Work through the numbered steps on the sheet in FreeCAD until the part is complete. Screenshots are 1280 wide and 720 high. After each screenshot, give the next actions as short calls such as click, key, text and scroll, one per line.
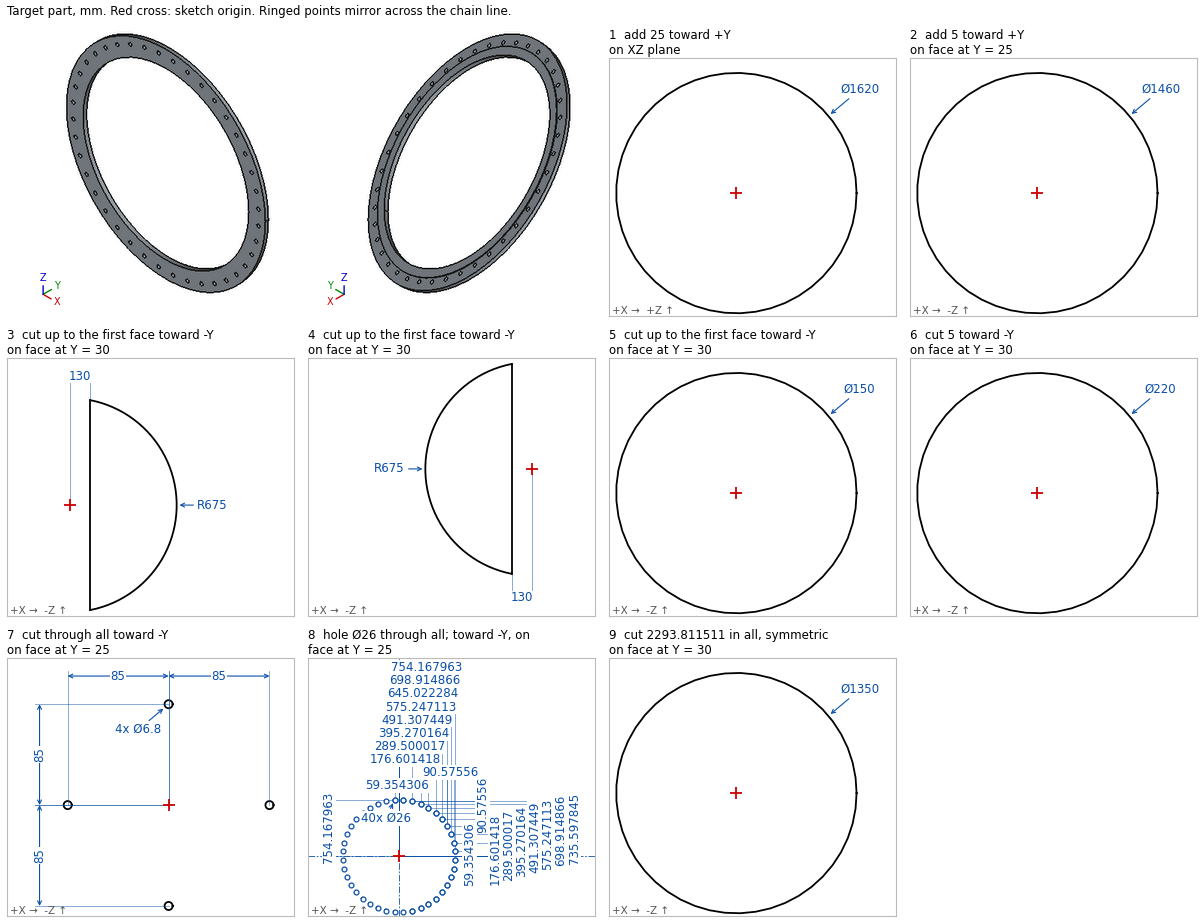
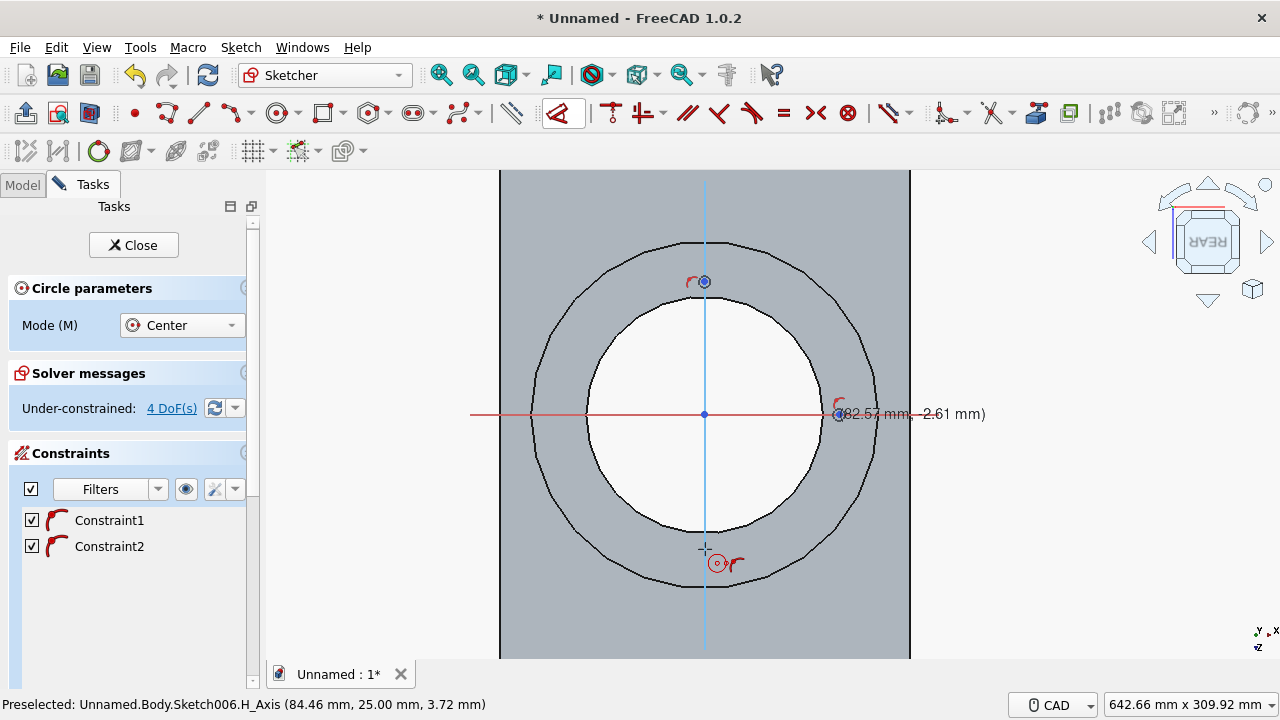
click(705, 549)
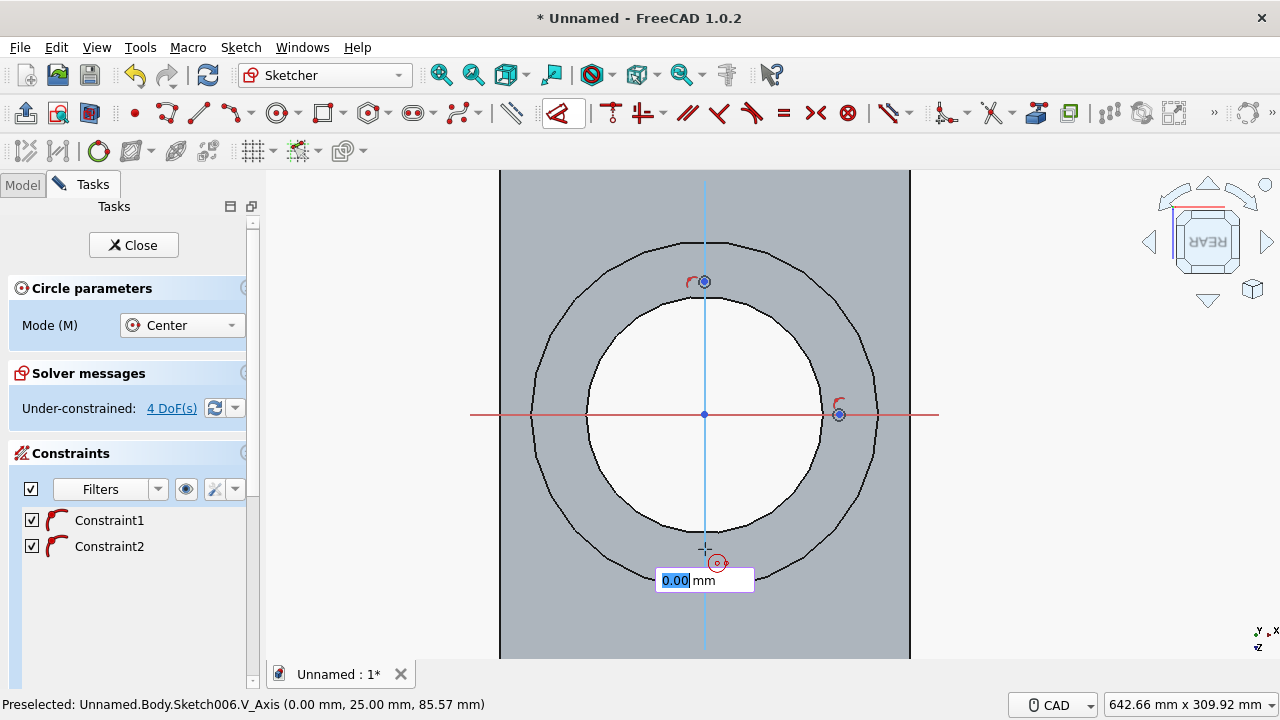
scroll(710, 547, up, 6)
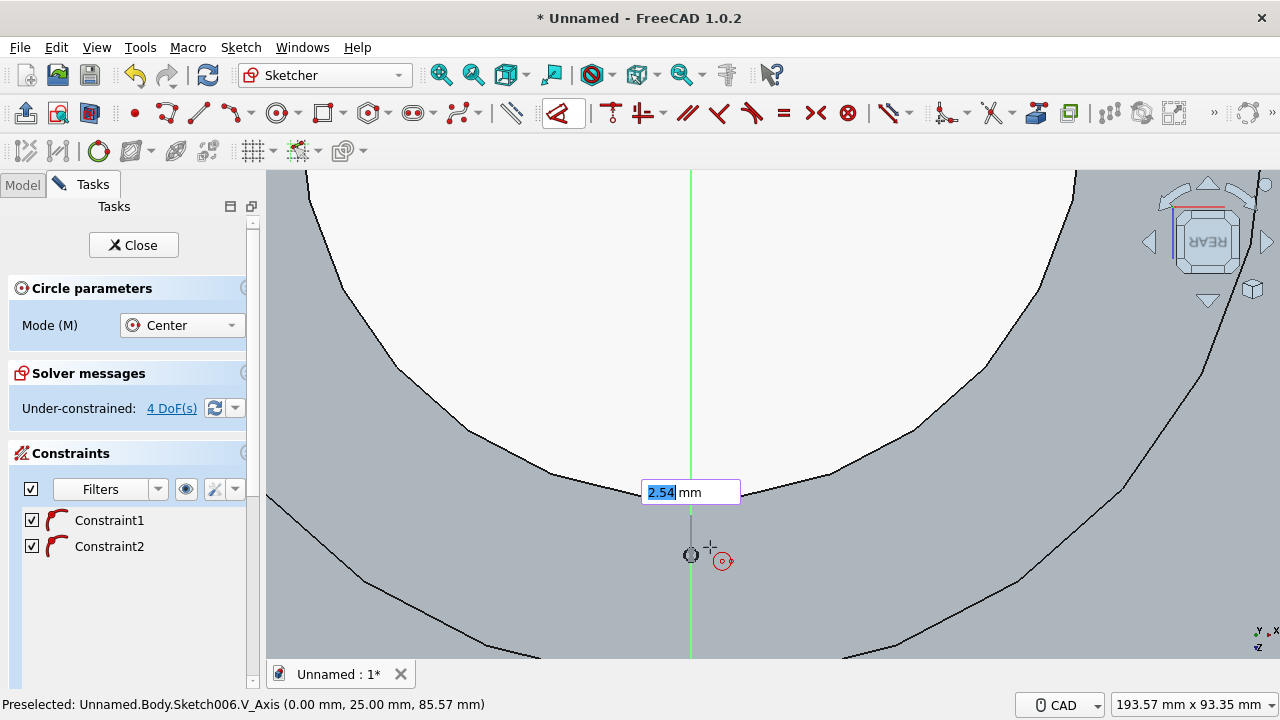
click(708, 546)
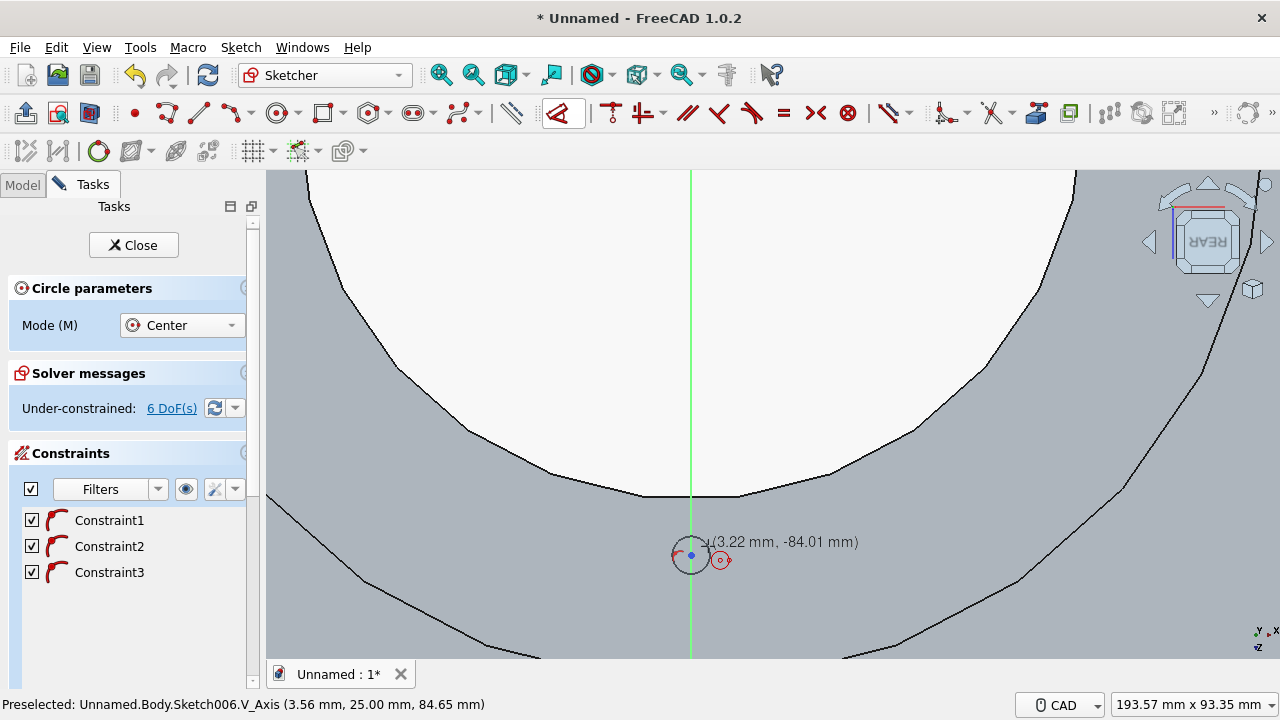
scroll(710, 547, down, 6)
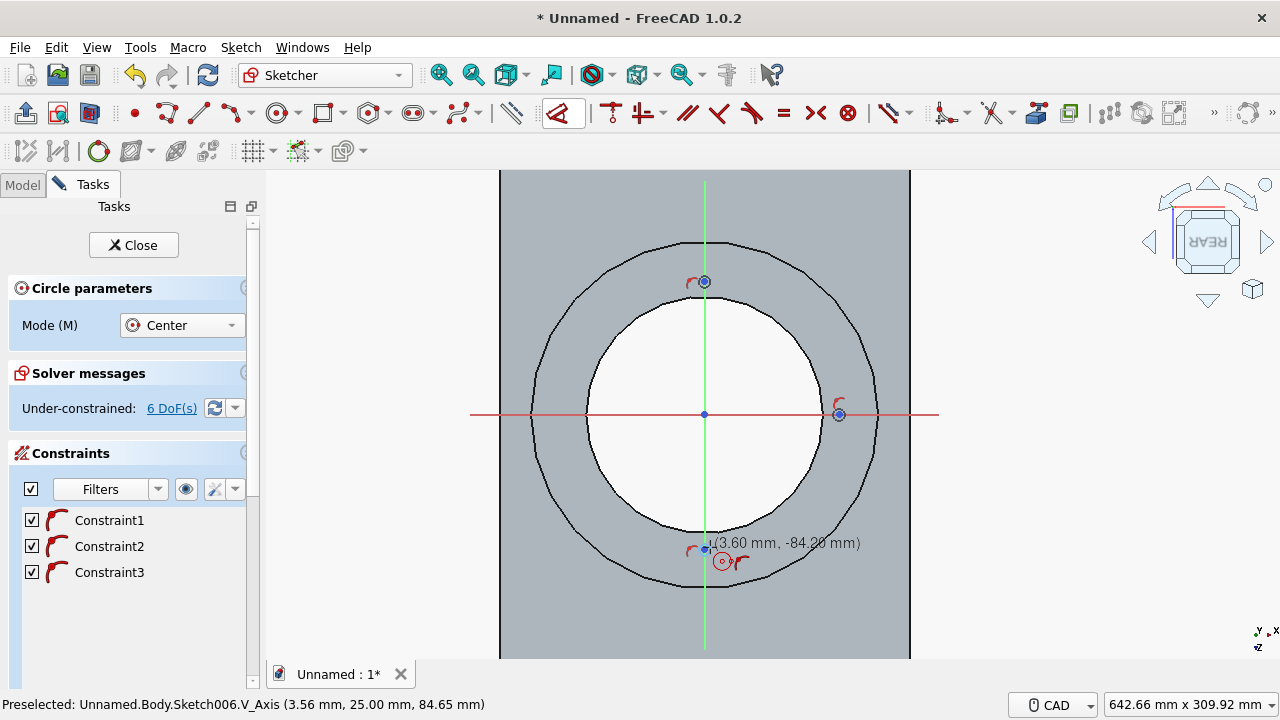
scroll(571, 415, up, 8)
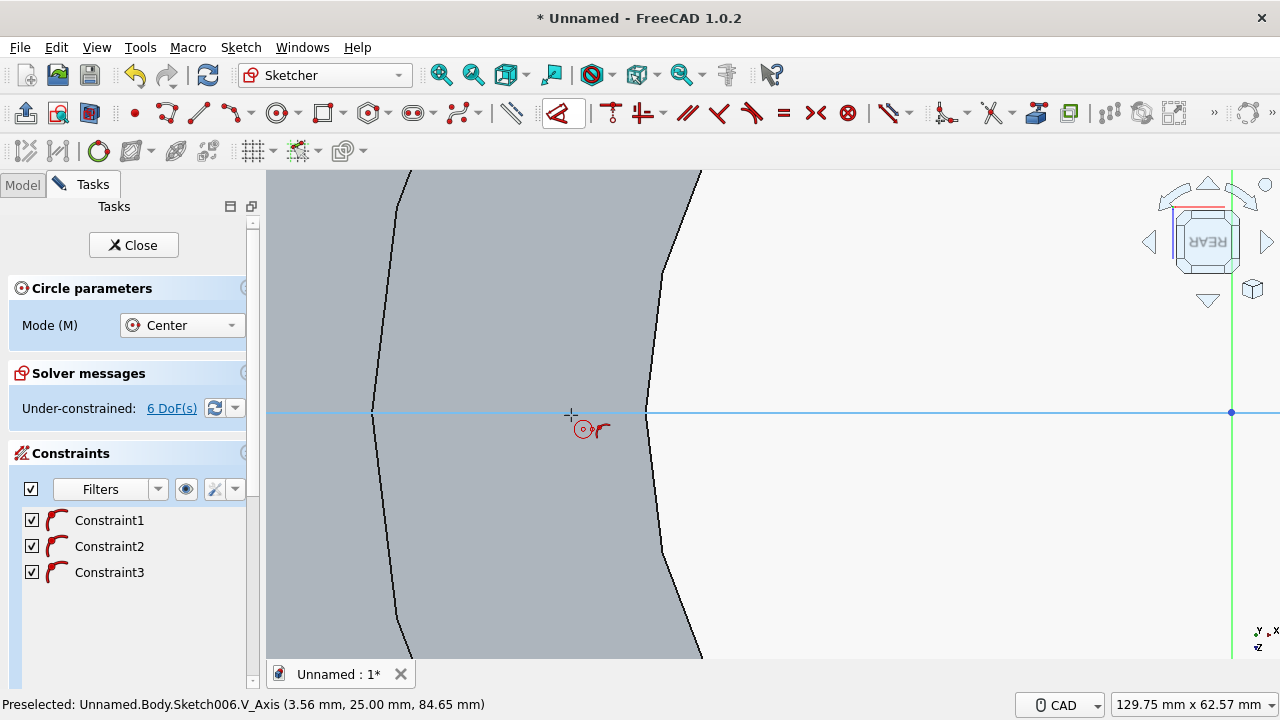
scroll(571, 415, down, 8)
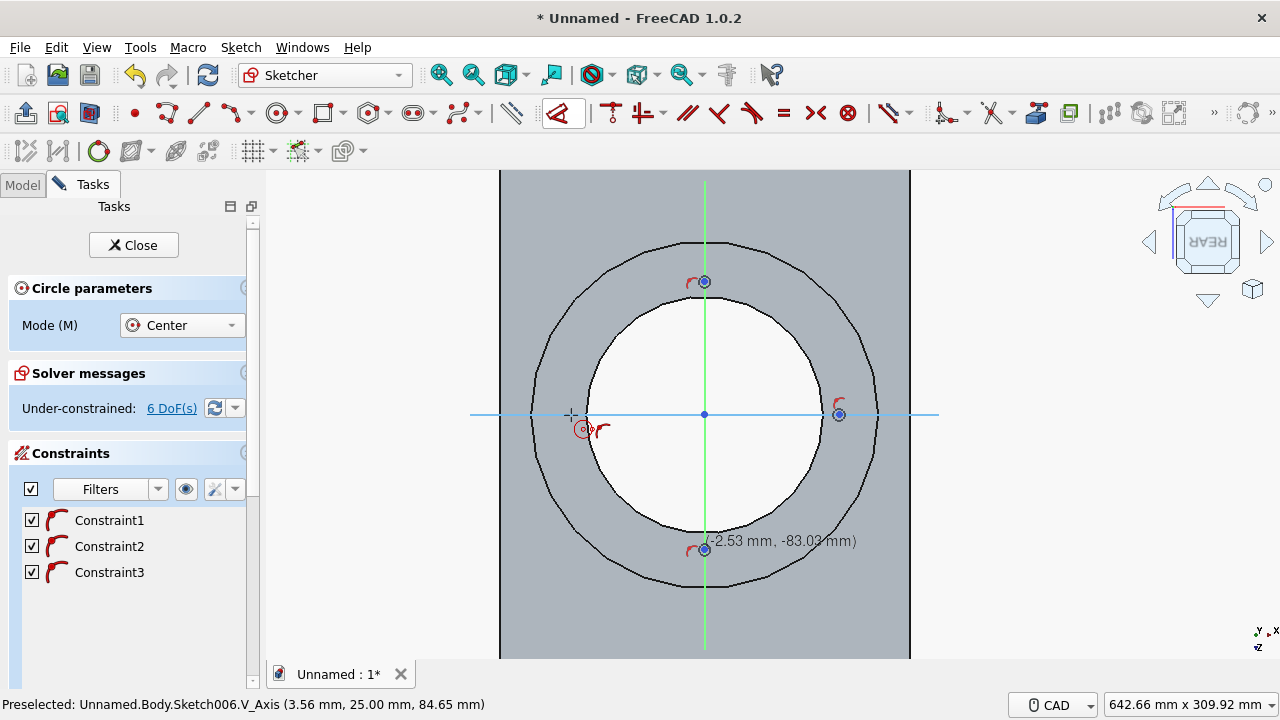
click(571, 415)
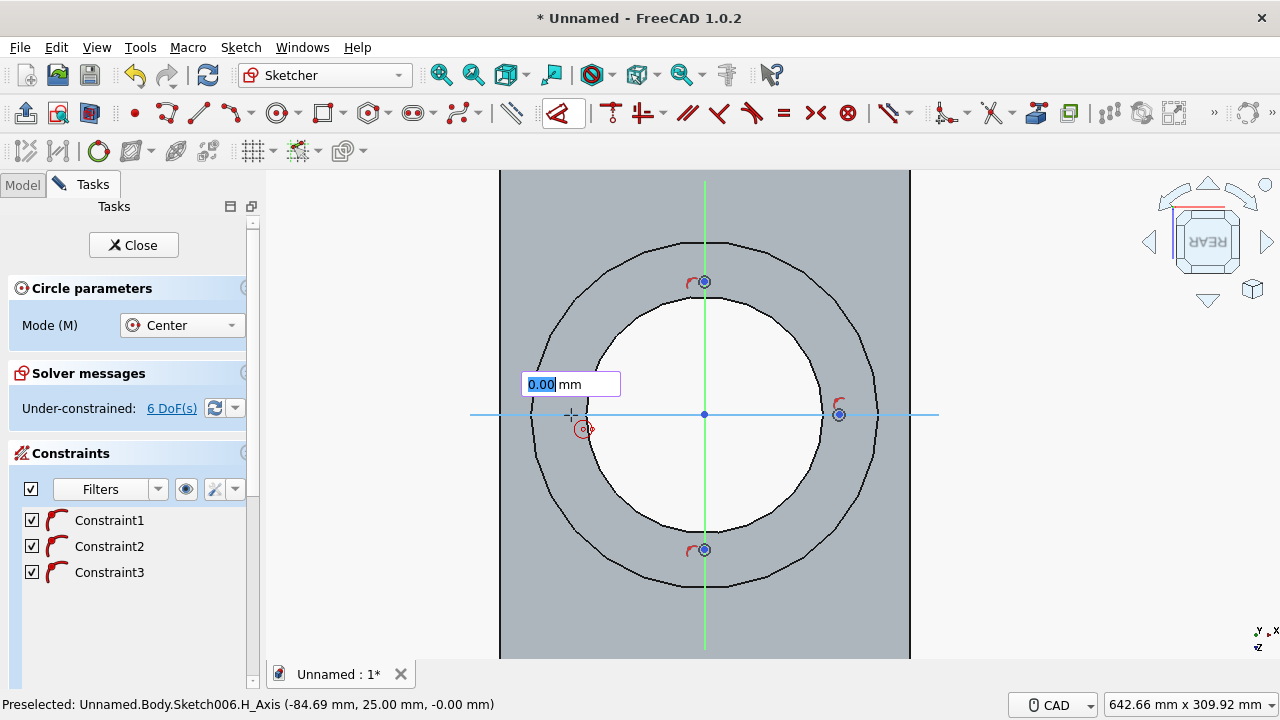
scroll(569, 420, up, 6)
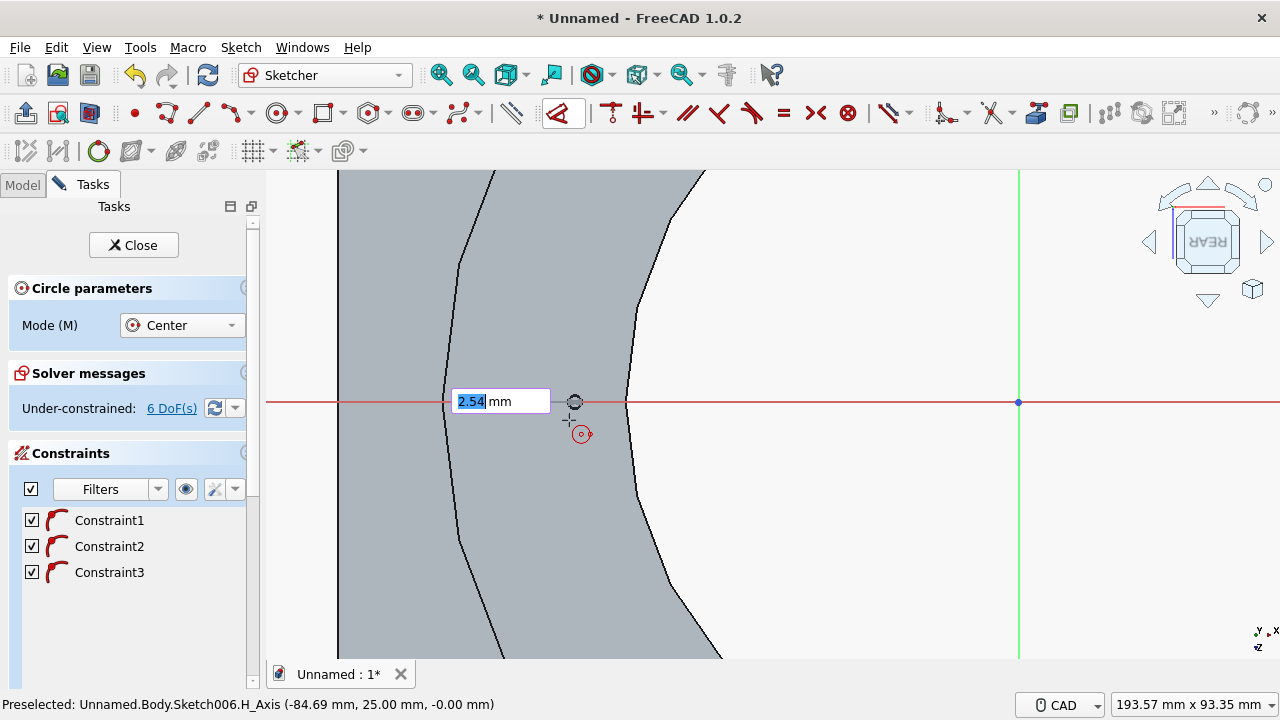
click(567, 419)
key(Escape)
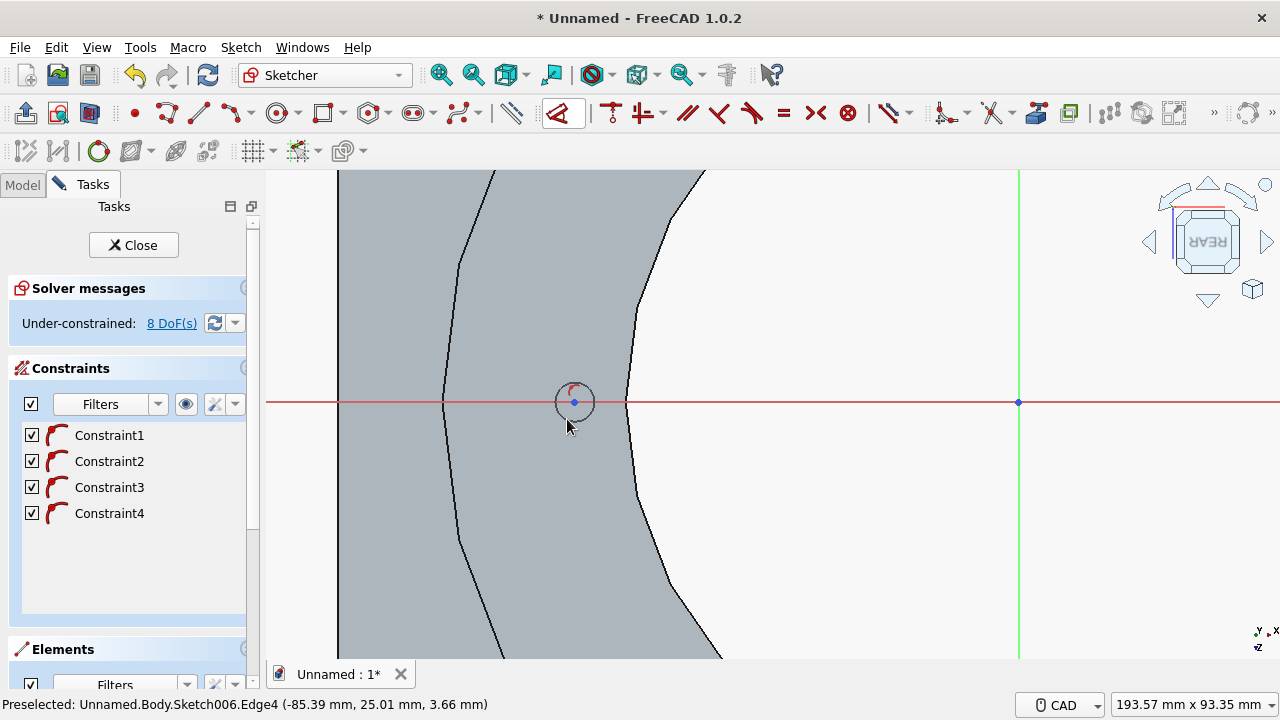
scroll(569, 420, down, 6)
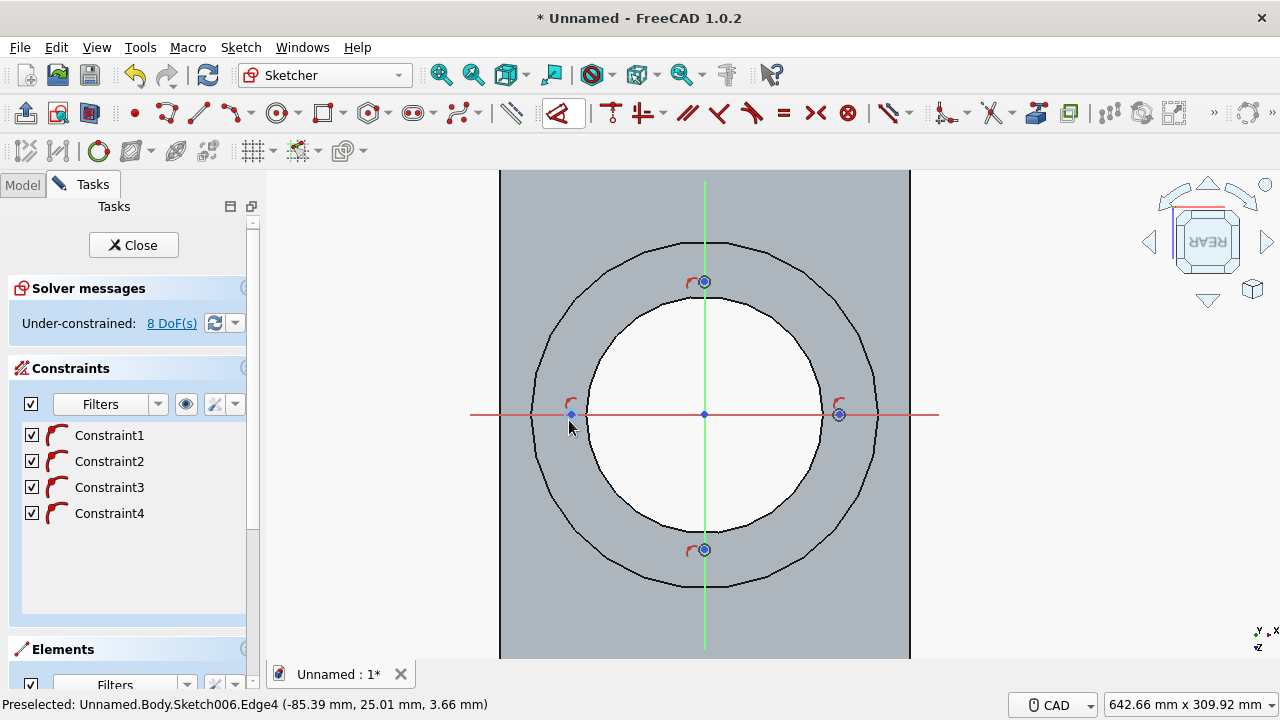
scroll(709, 278, up, 7)